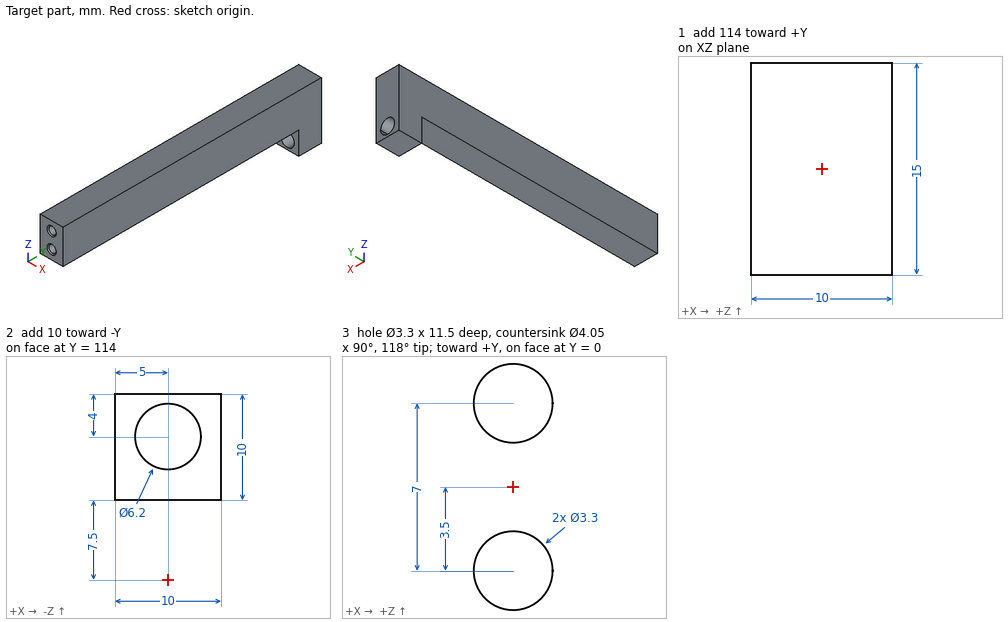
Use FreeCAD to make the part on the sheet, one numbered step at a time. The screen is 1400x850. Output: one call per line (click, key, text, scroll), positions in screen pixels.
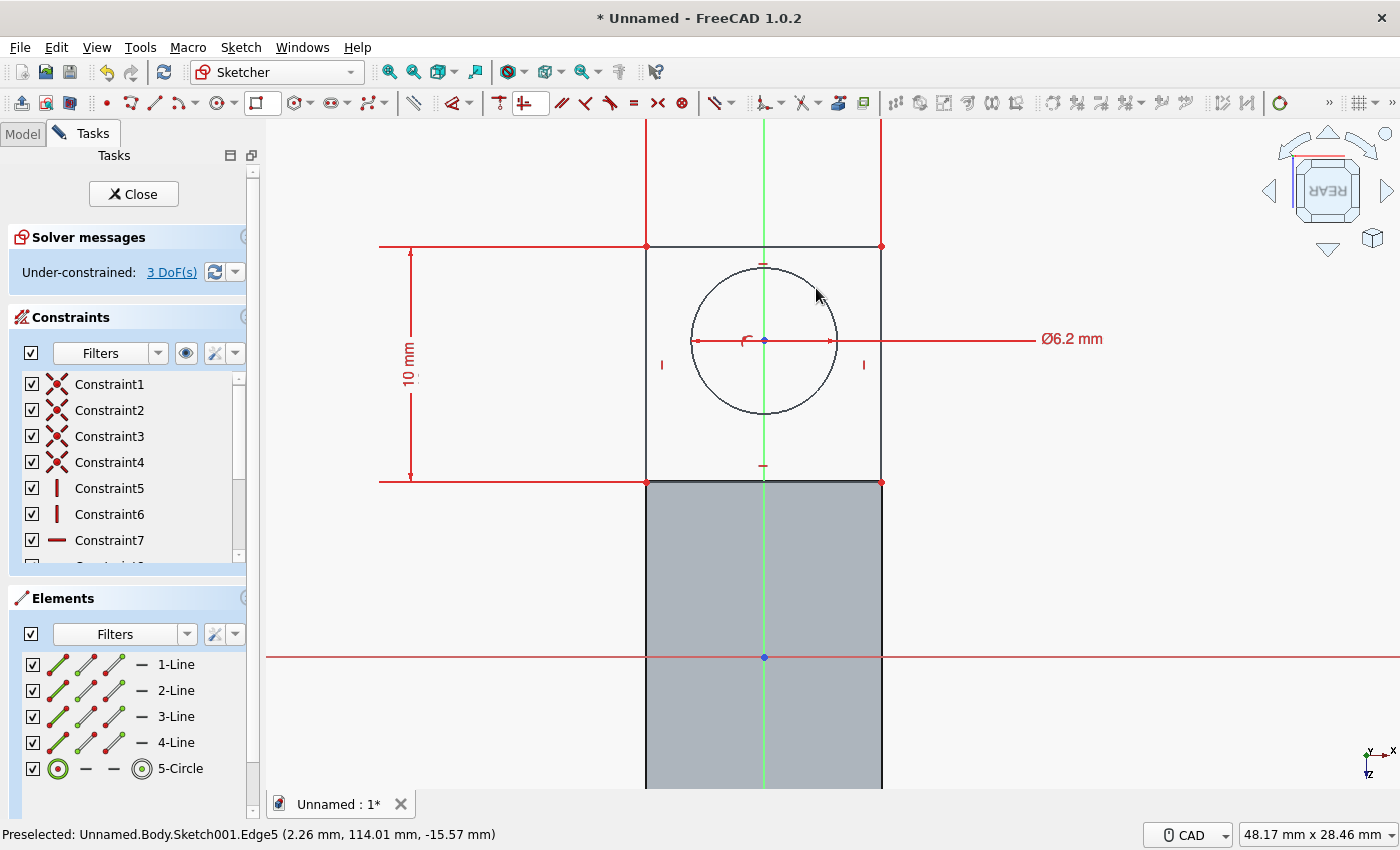
click(646, 247)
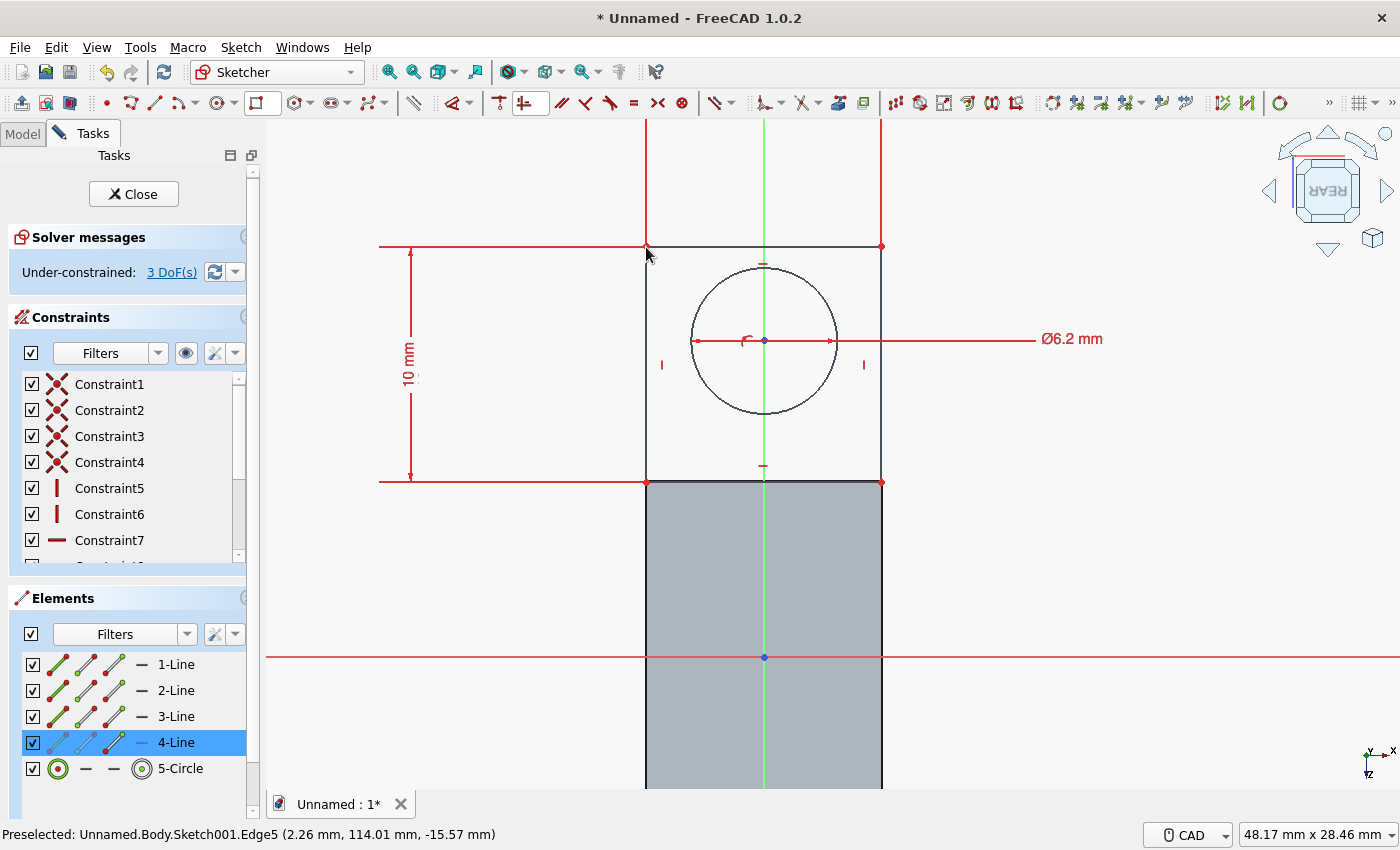
click(472, 104)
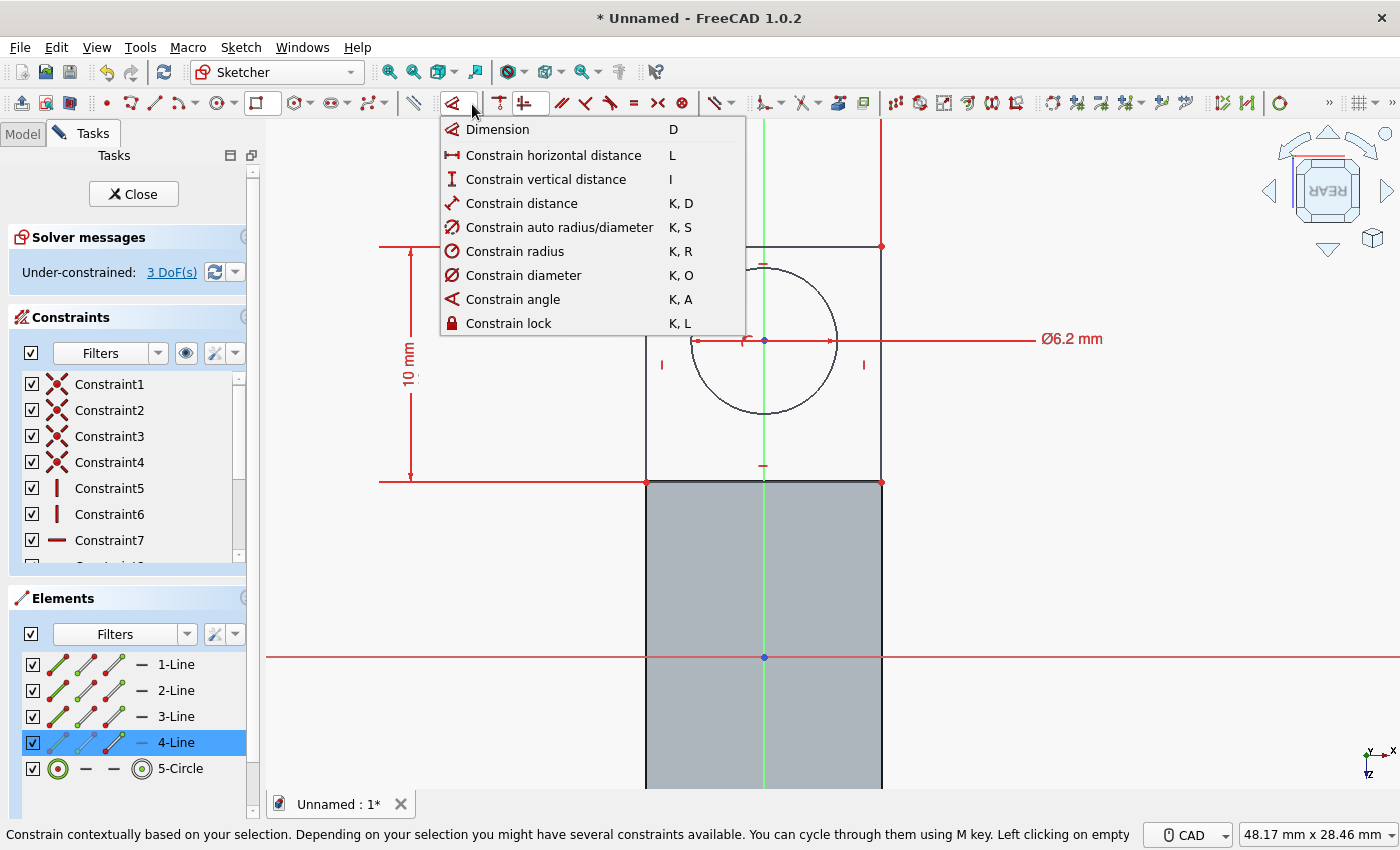
click(593, 155)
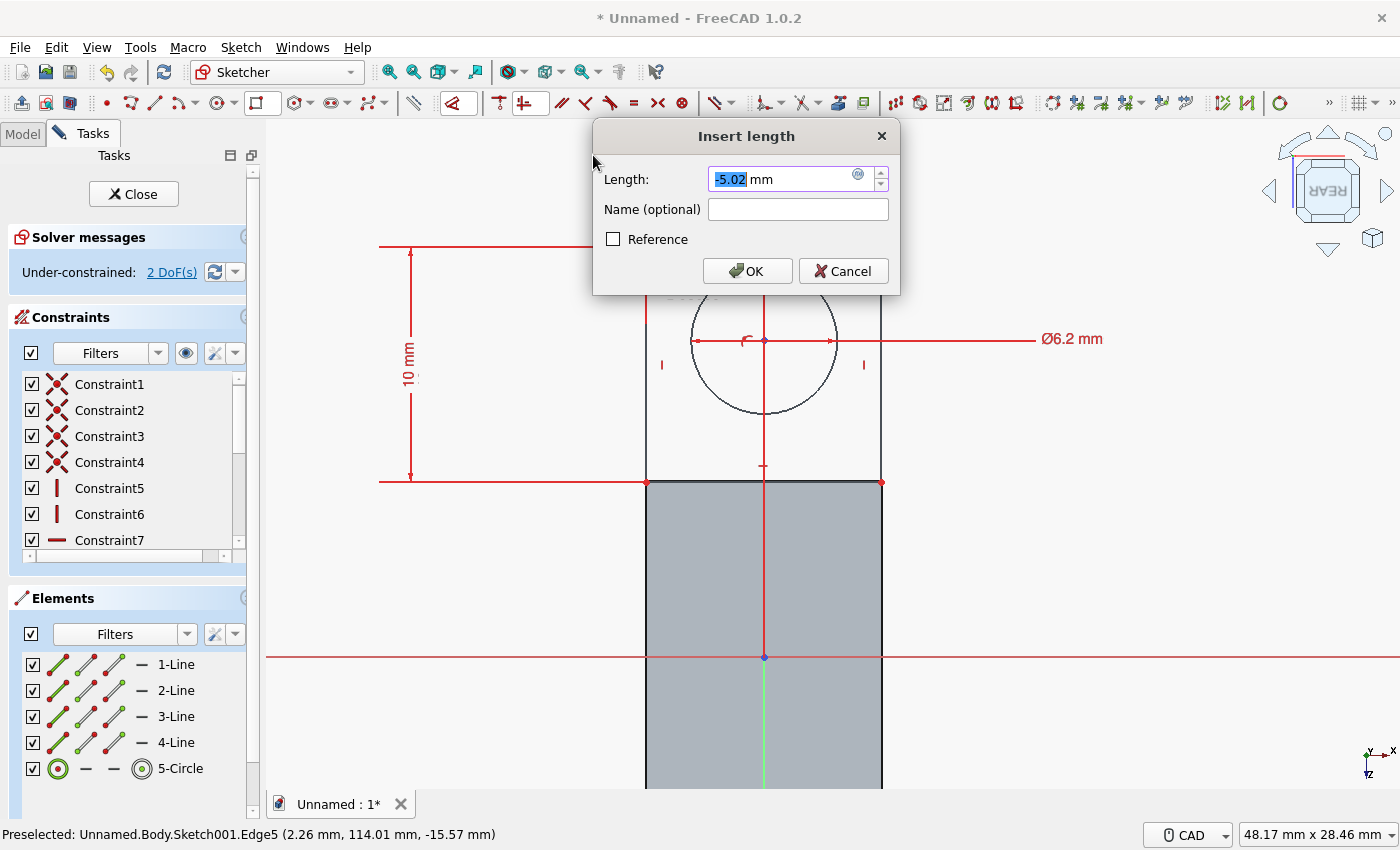
text(-5)
key(Return)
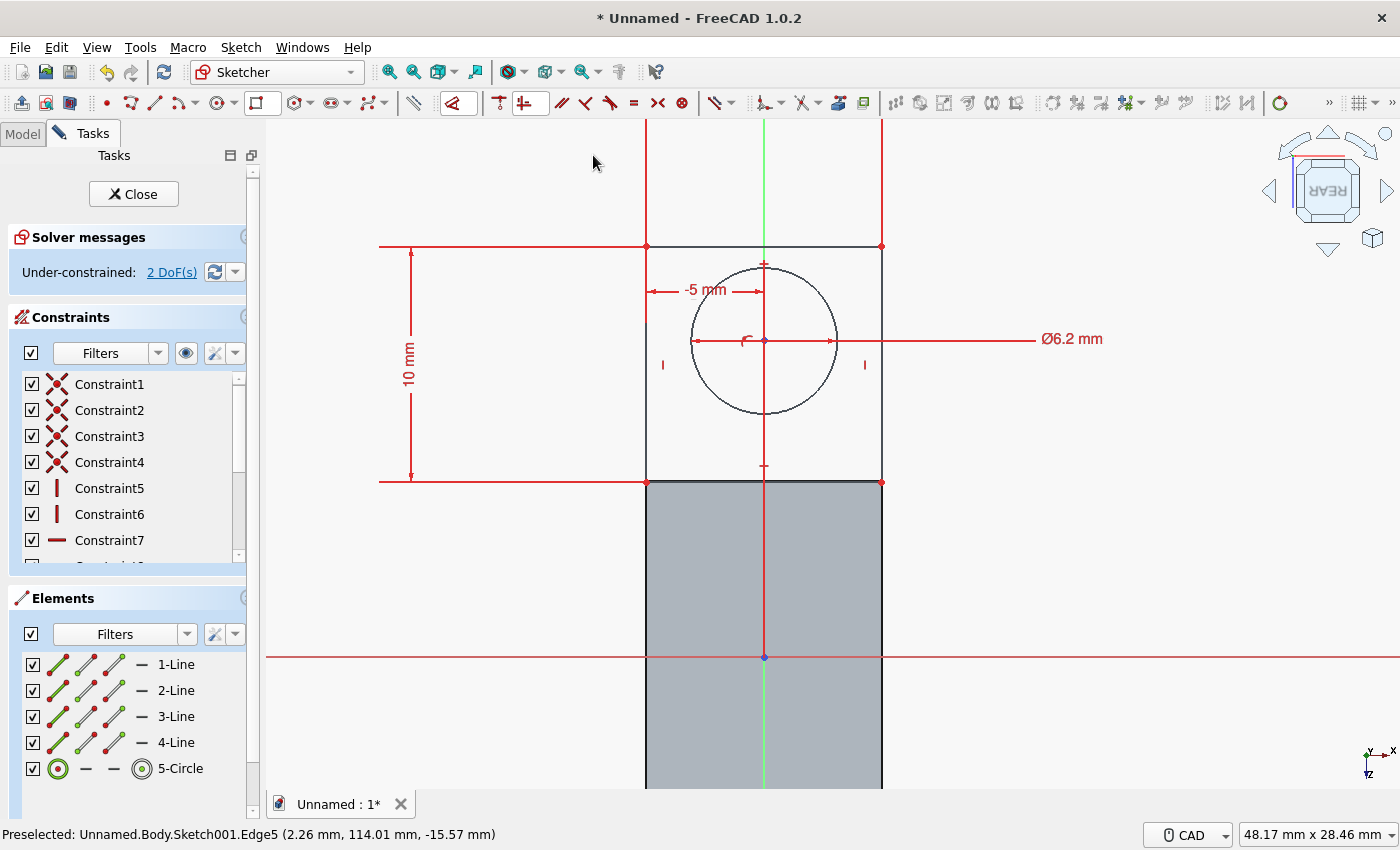
click(646, 247)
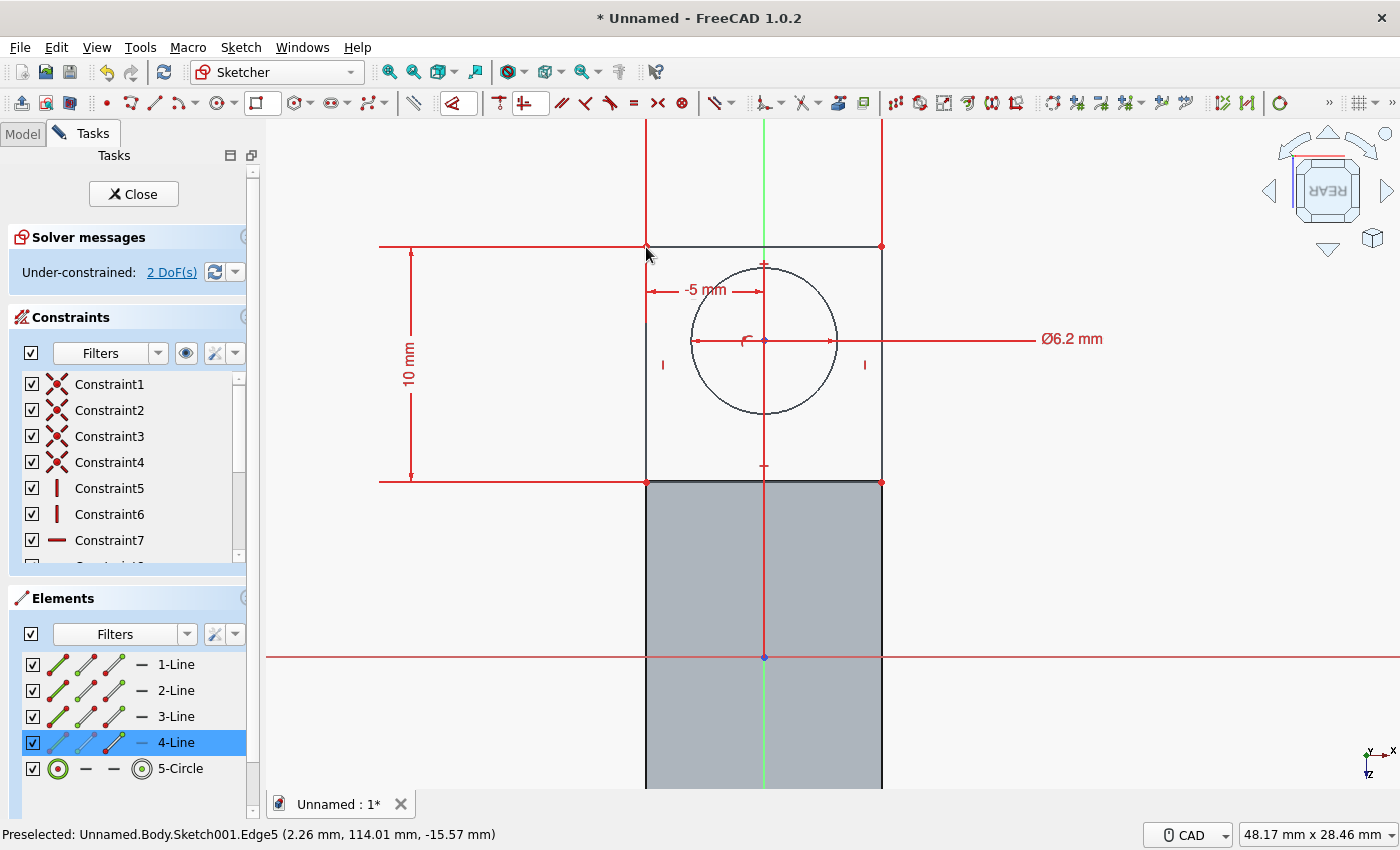
scroll(764, 341, up, 4)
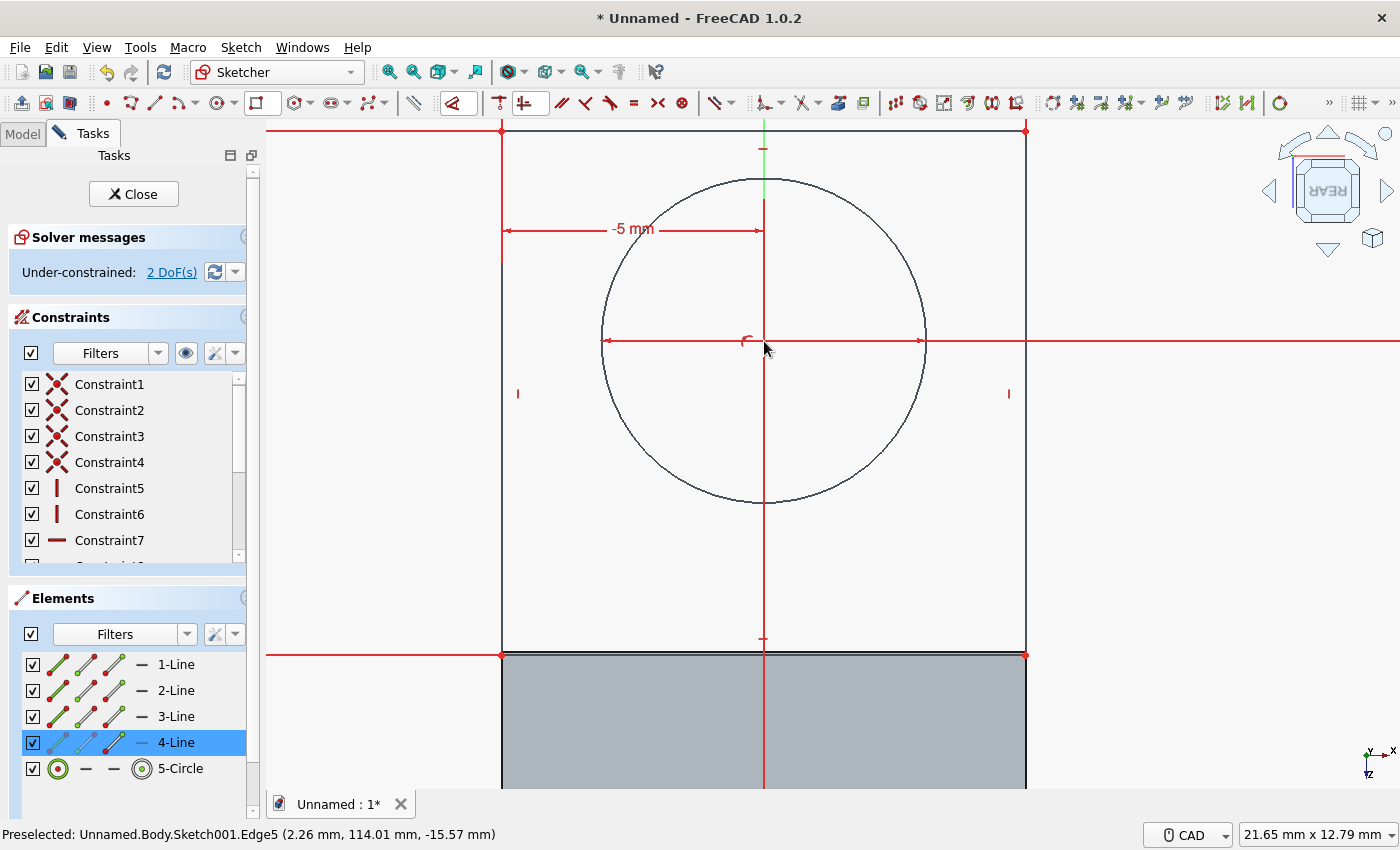
click(764, 341)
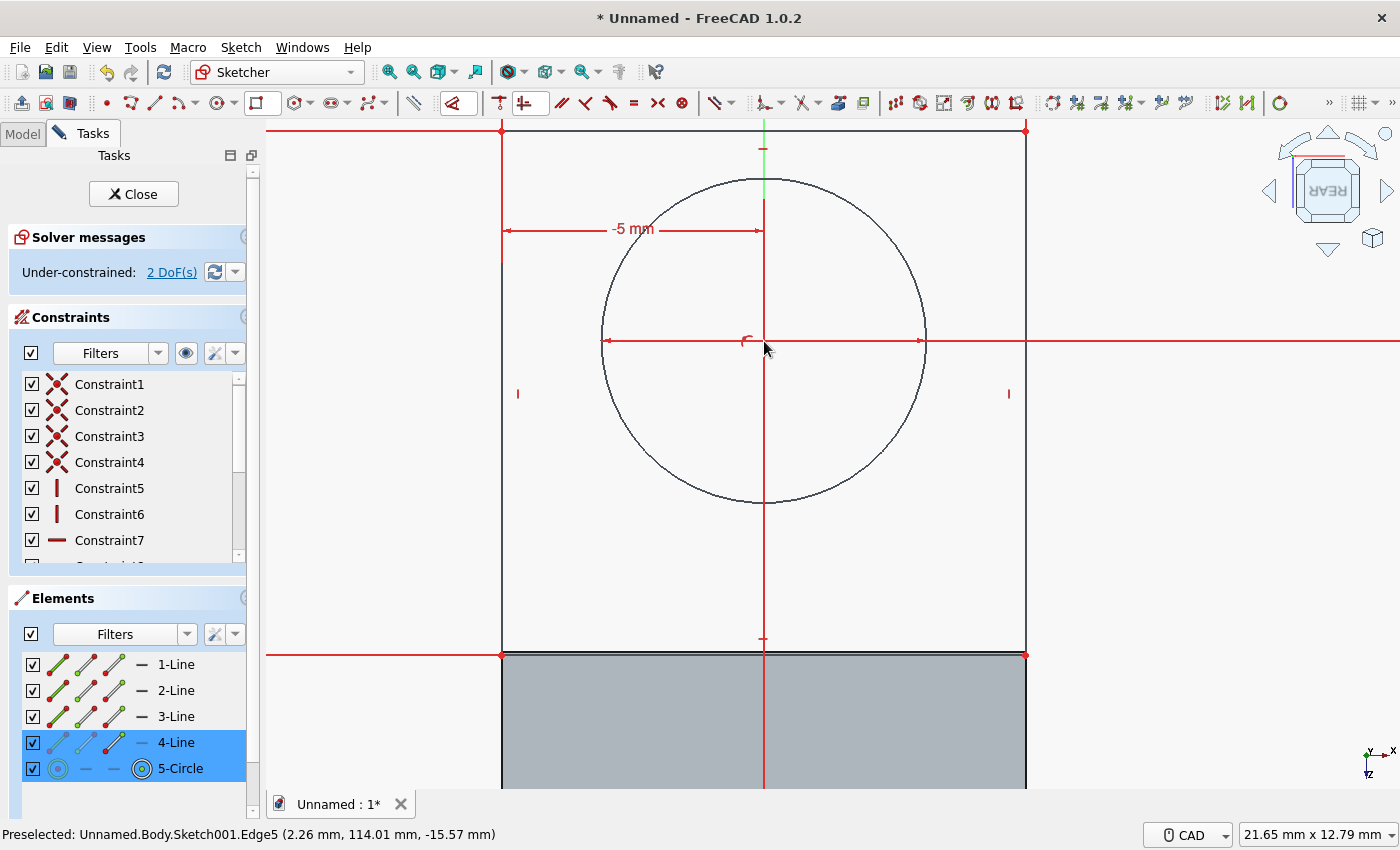
key(i)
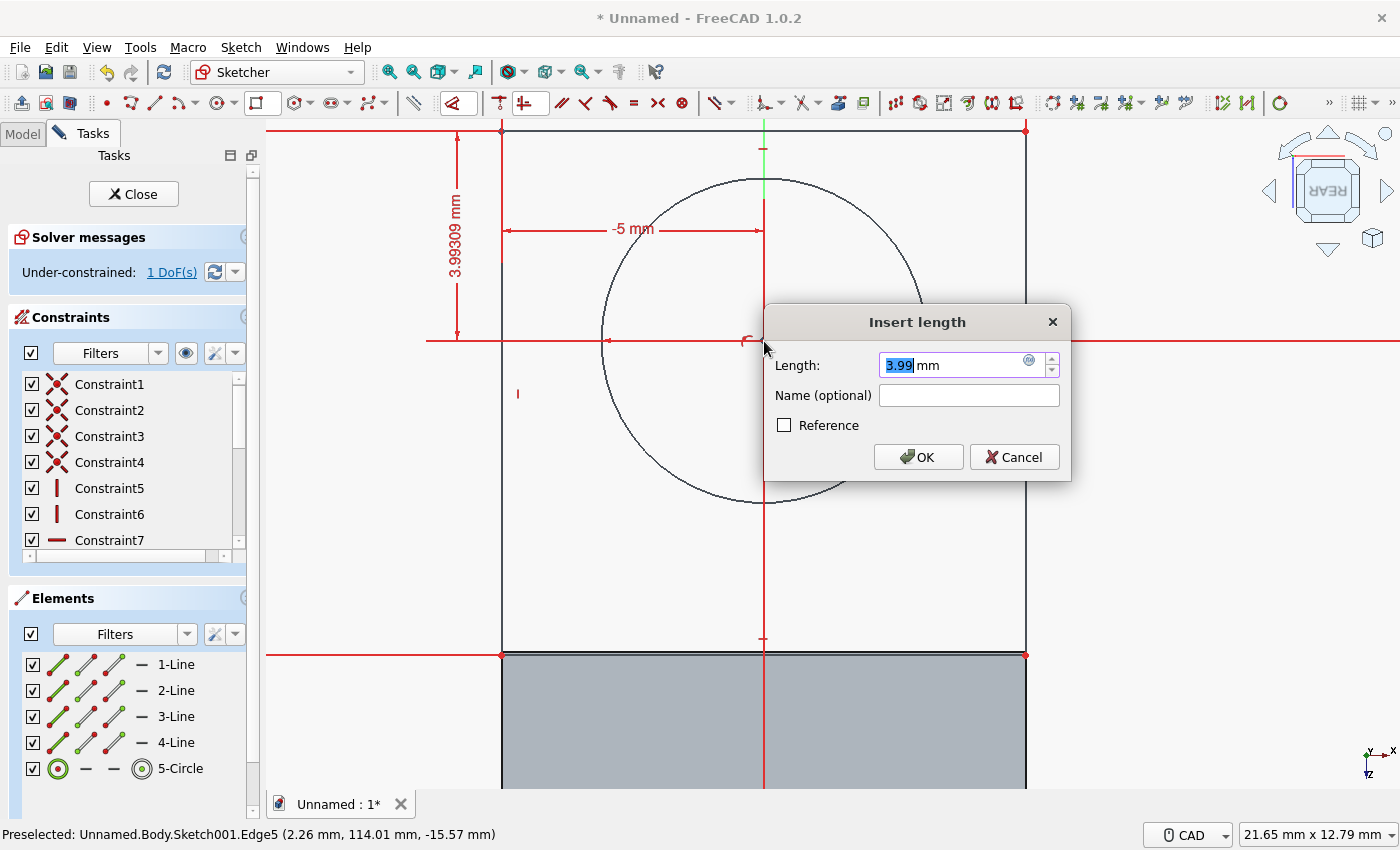
text(4)
key(Return)